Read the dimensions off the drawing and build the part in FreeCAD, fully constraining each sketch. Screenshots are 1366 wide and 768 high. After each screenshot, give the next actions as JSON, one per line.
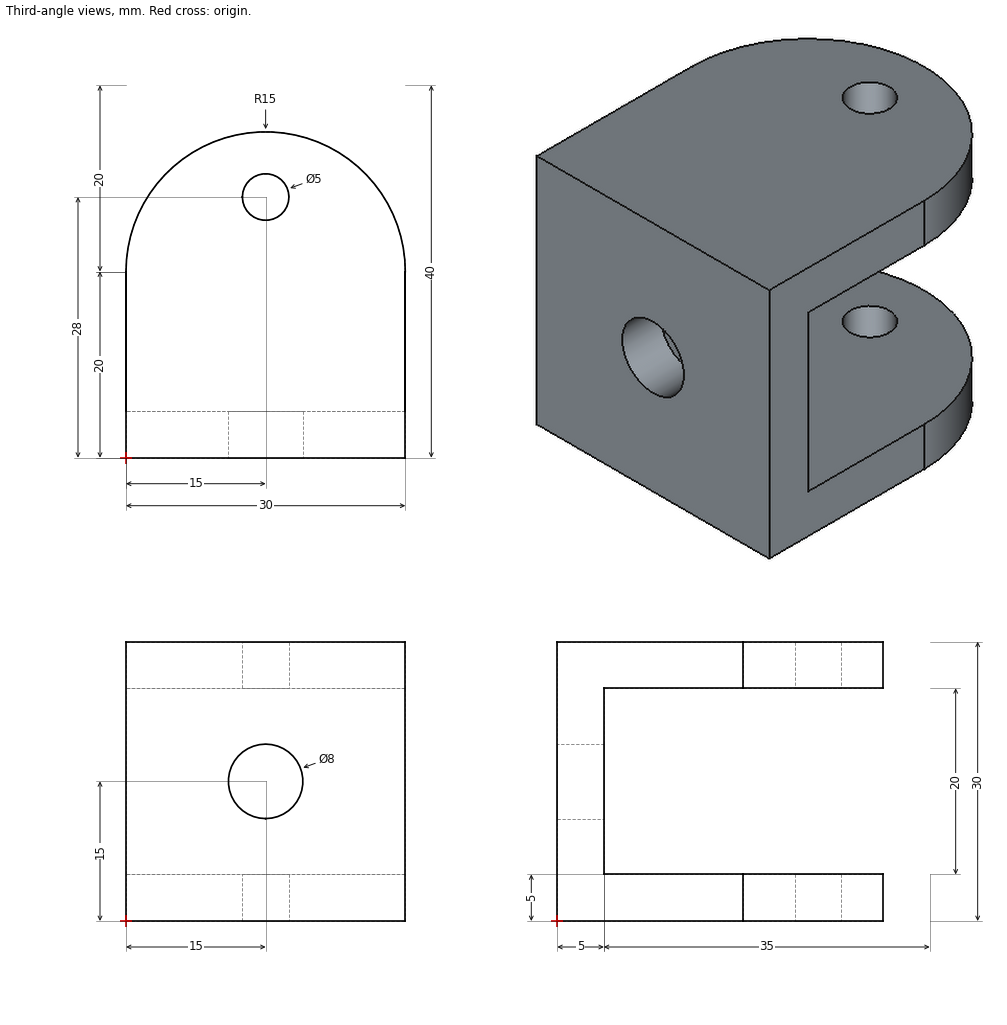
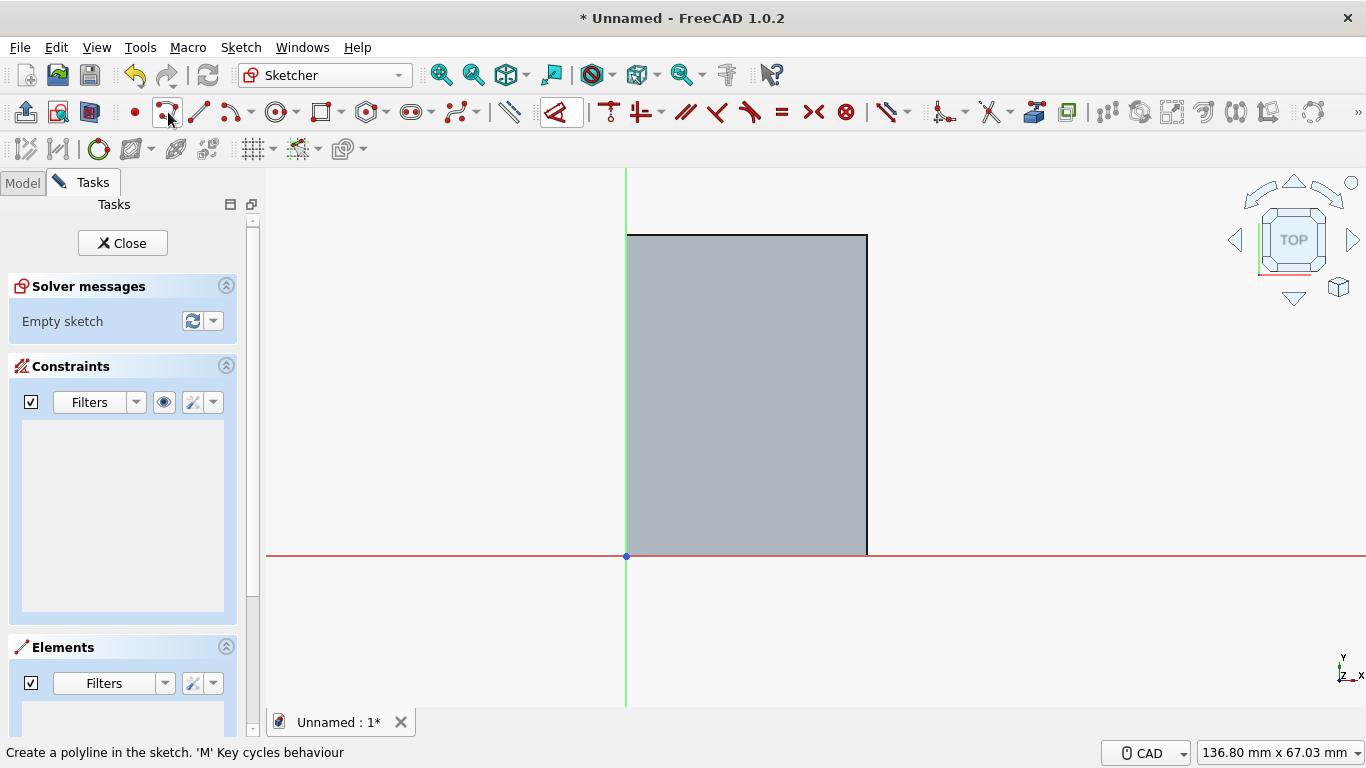
{"action": "left_click", "coordinate": [626, 395]}
{"action": "left_click", "coordinate": [635, 235]}
{"action": "left_click", "coordinate": [867, 235]}
{"action": "left_click", "coordinate": [867, 395]}
{"action": "right_click", "coordinate": [867, 395]}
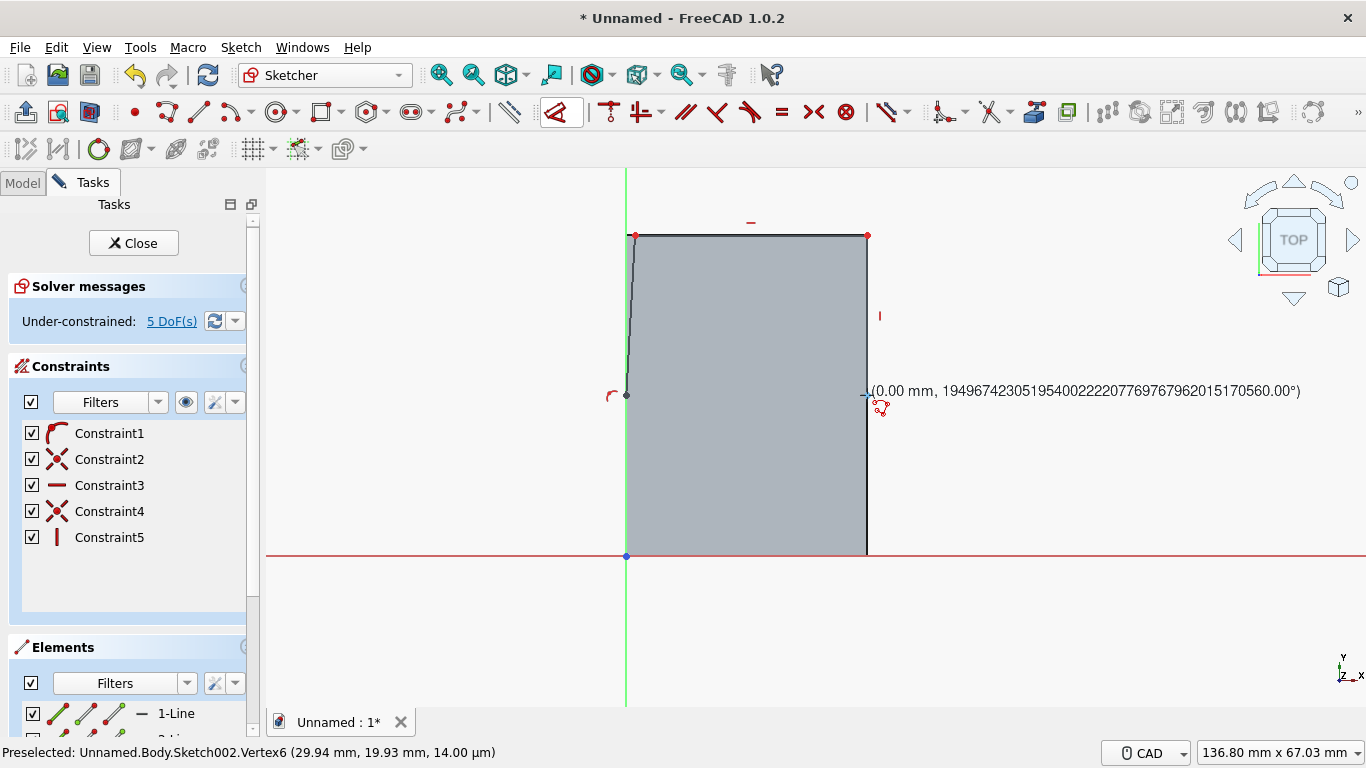
{"action": "left_click", "coordinate": [254, 112]}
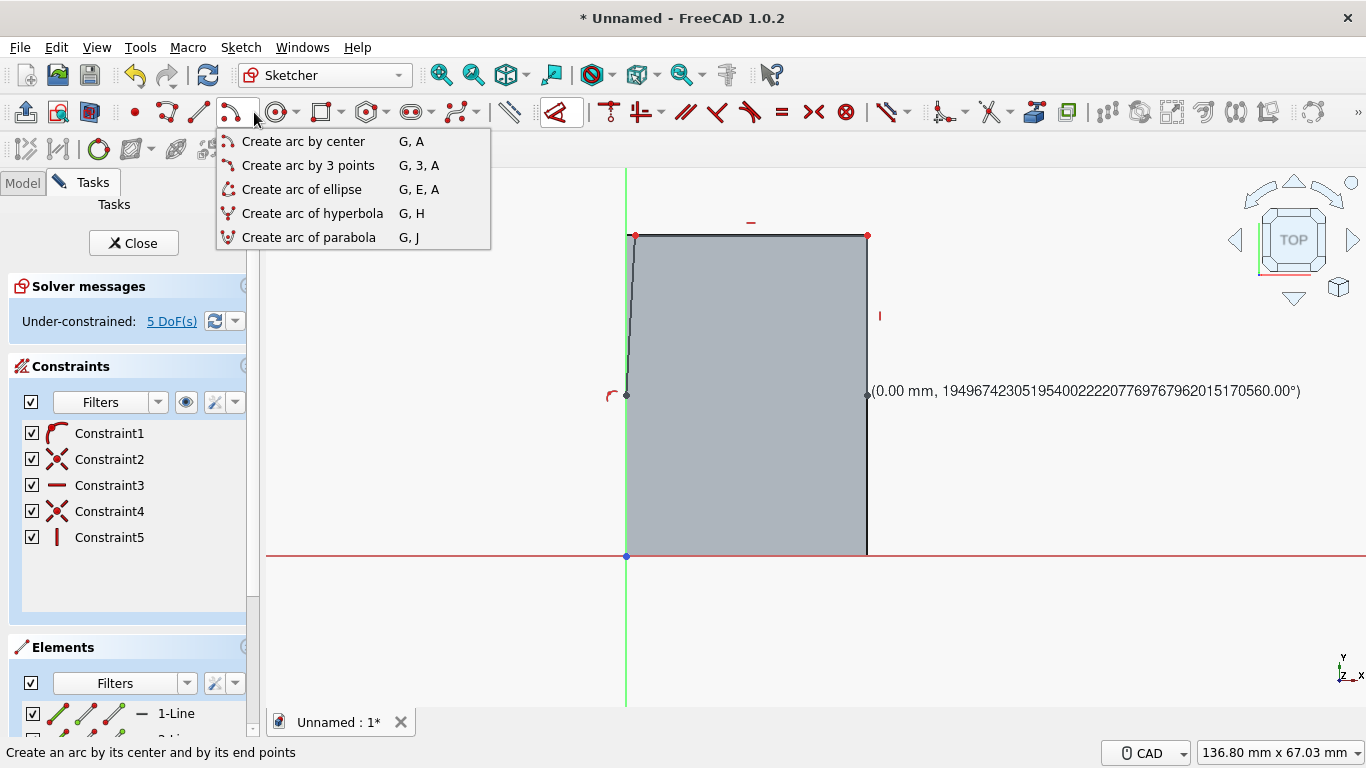
{"action": "left_click", "coordinate": [354, 165]}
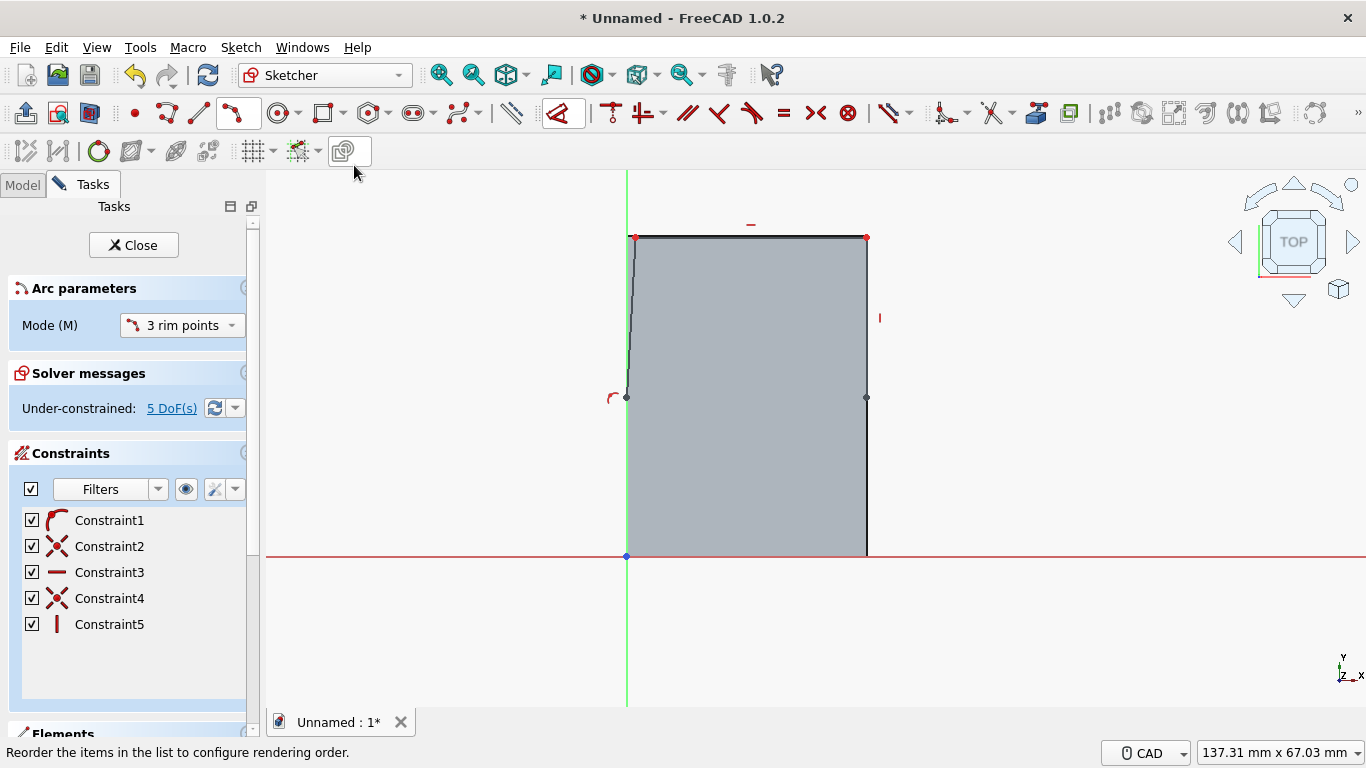
{"action": "left_click", "coordinate": [867, 397]}
{"action": "left_click", "coordinate": [627, 397]}
{"action": "left_click", "coordinate": [747, 276]}
{"action": "key", "text": "Escape"}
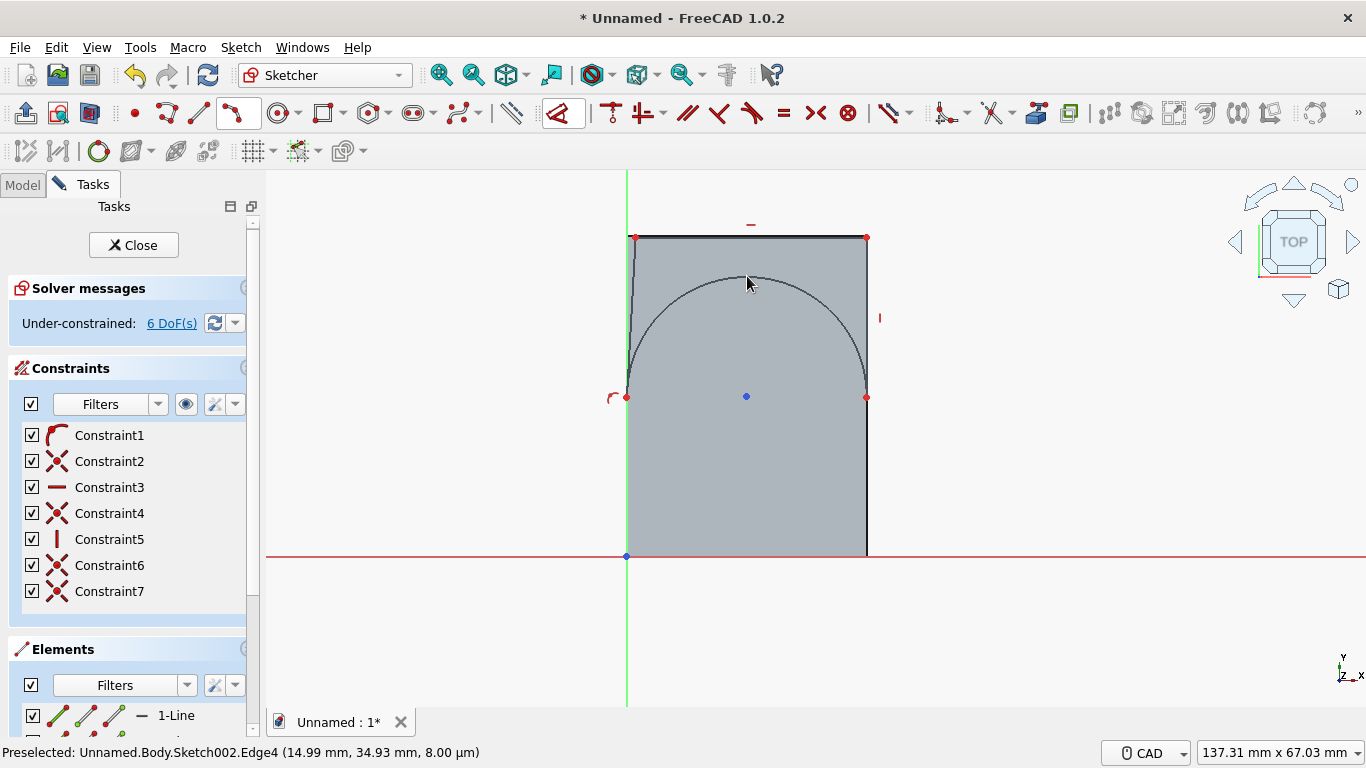
{"action": "left_click", "coordinate": [630, 333]}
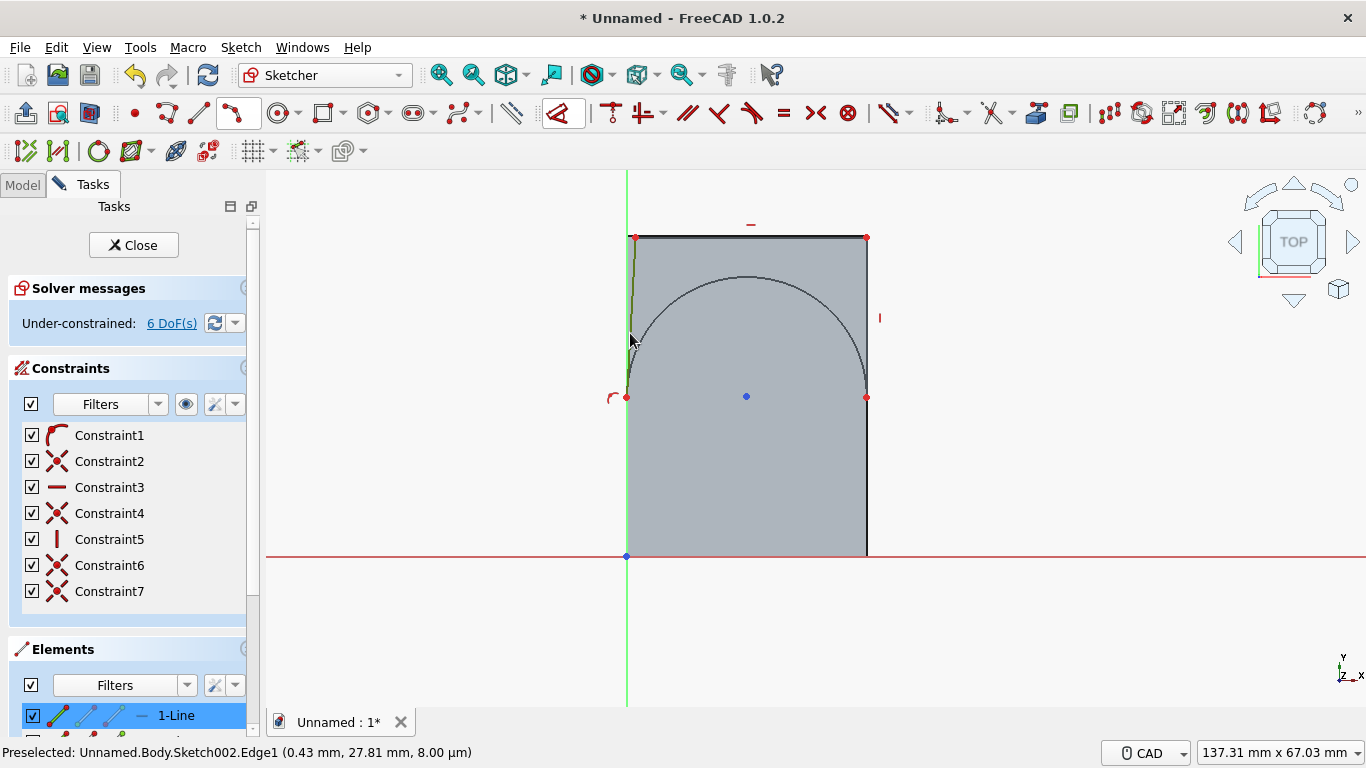
{"action": "left_click", "coordinate": [817, 300]}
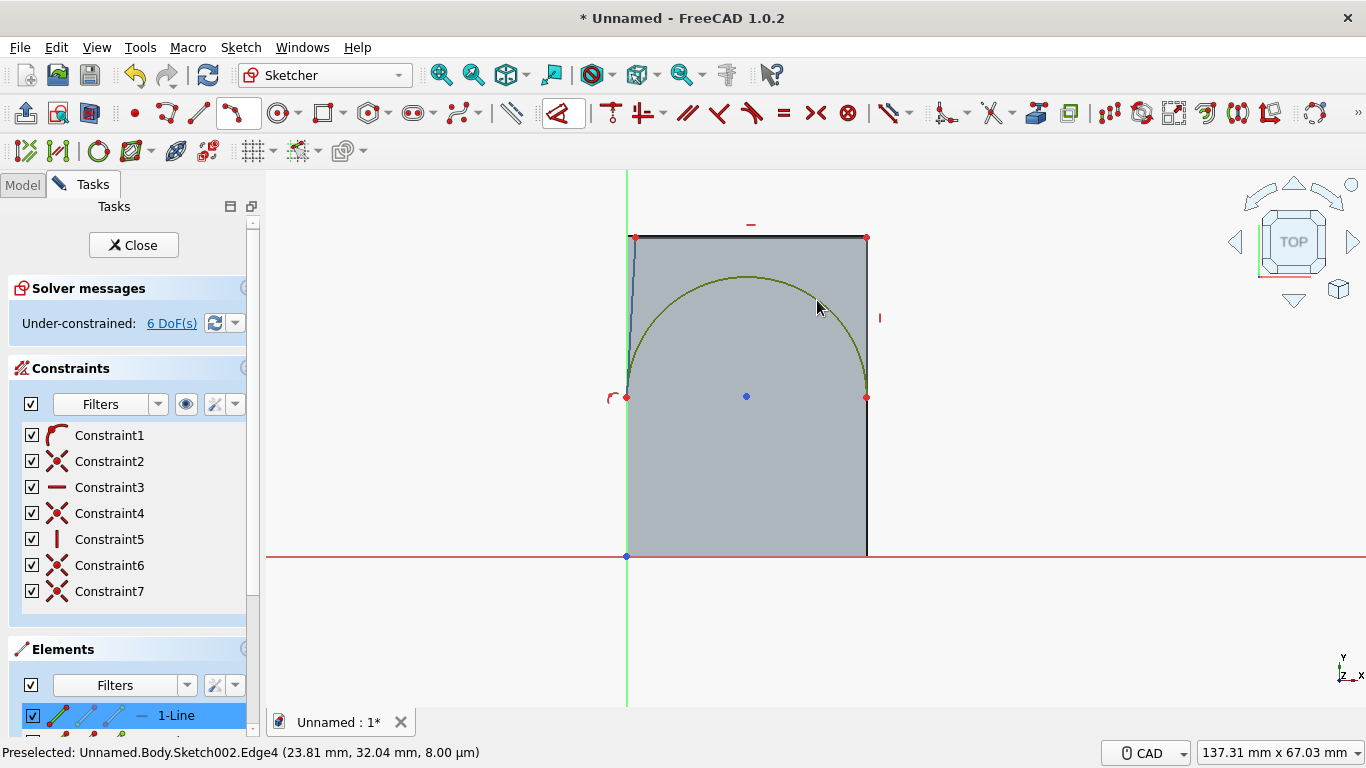
{"action": "left_click", "coordinate": [752, 114]}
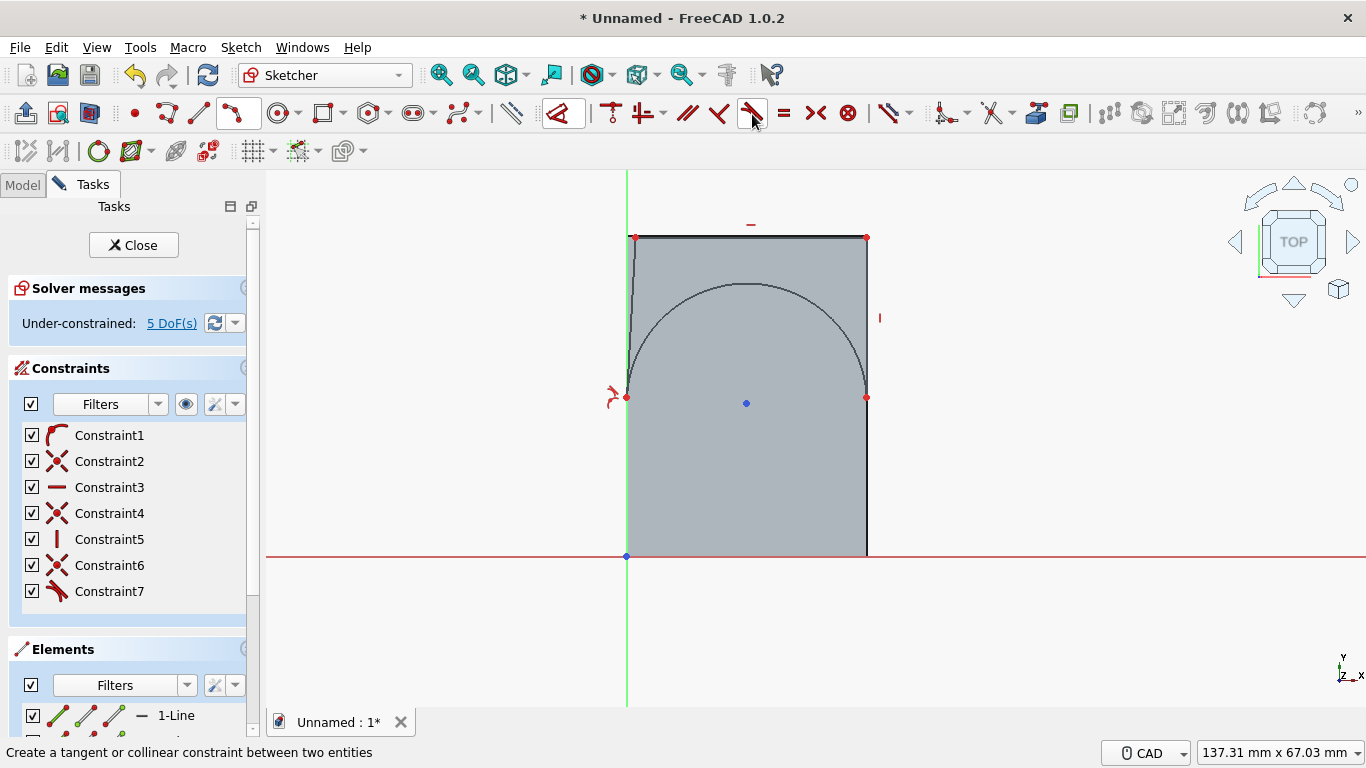
{"action": "left_click", "coordinate": [867, 286]}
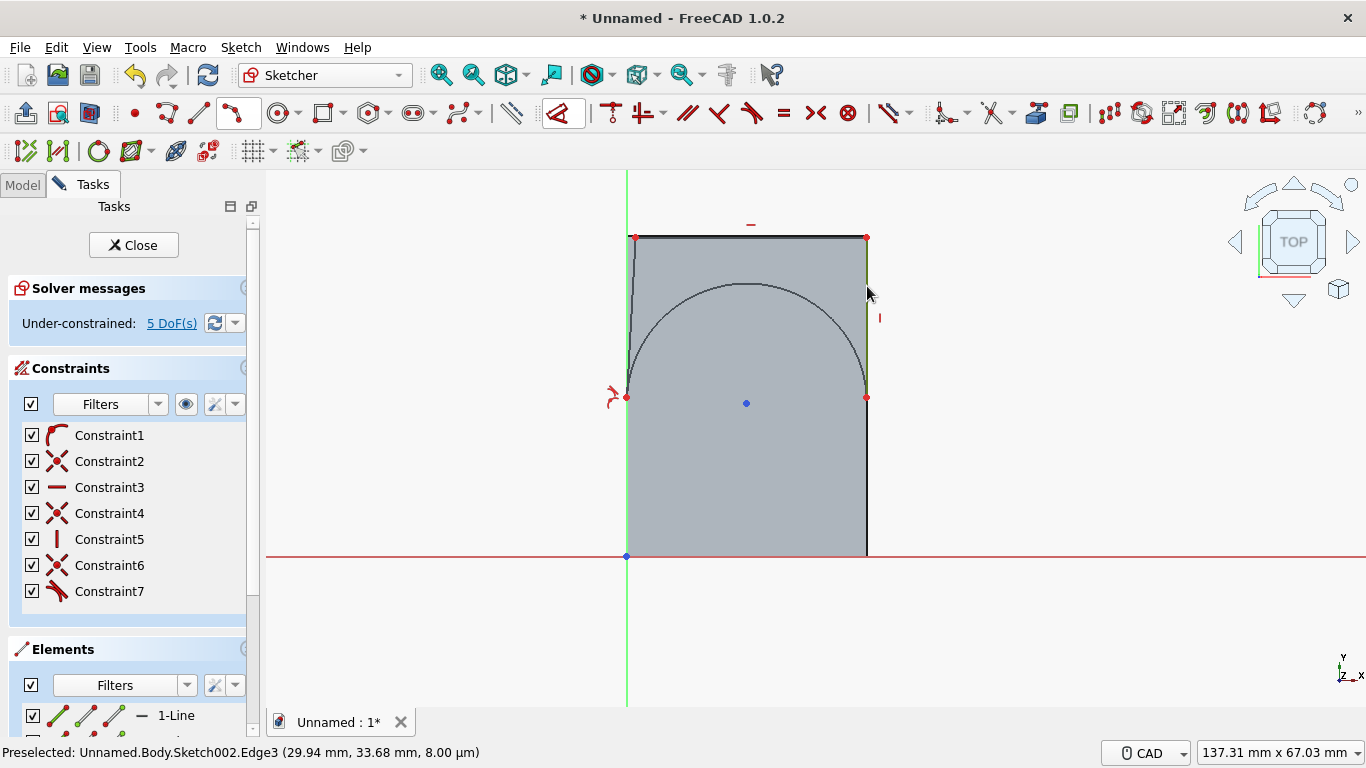
{"action": "left_click", "coordinate": [815, 305]}